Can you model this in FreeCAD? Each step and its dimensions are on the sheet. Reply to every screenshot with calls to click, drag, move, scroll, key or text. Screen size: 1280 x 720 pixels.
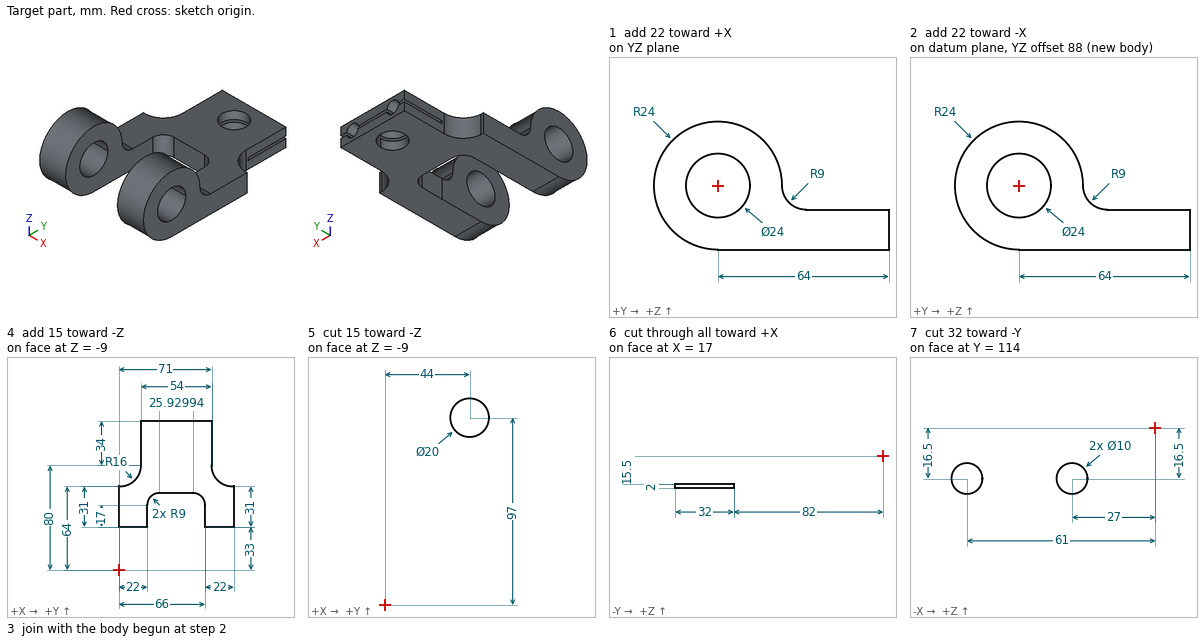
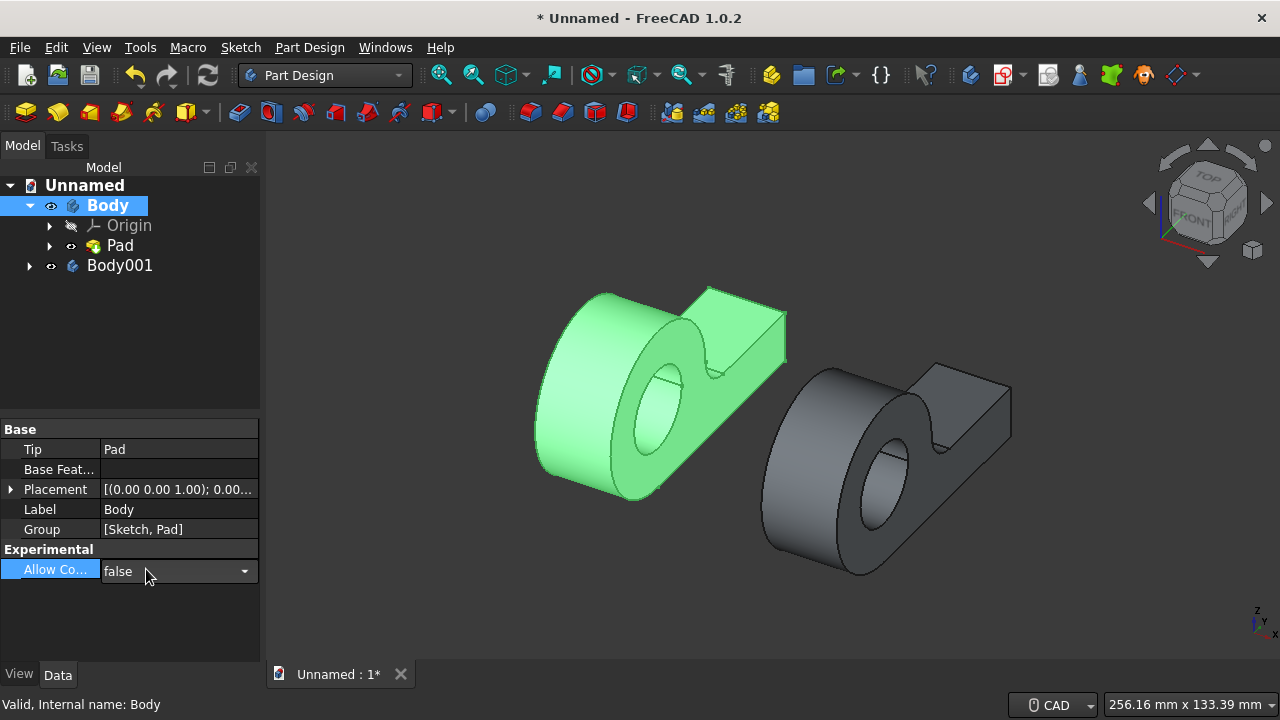
click(146, 569)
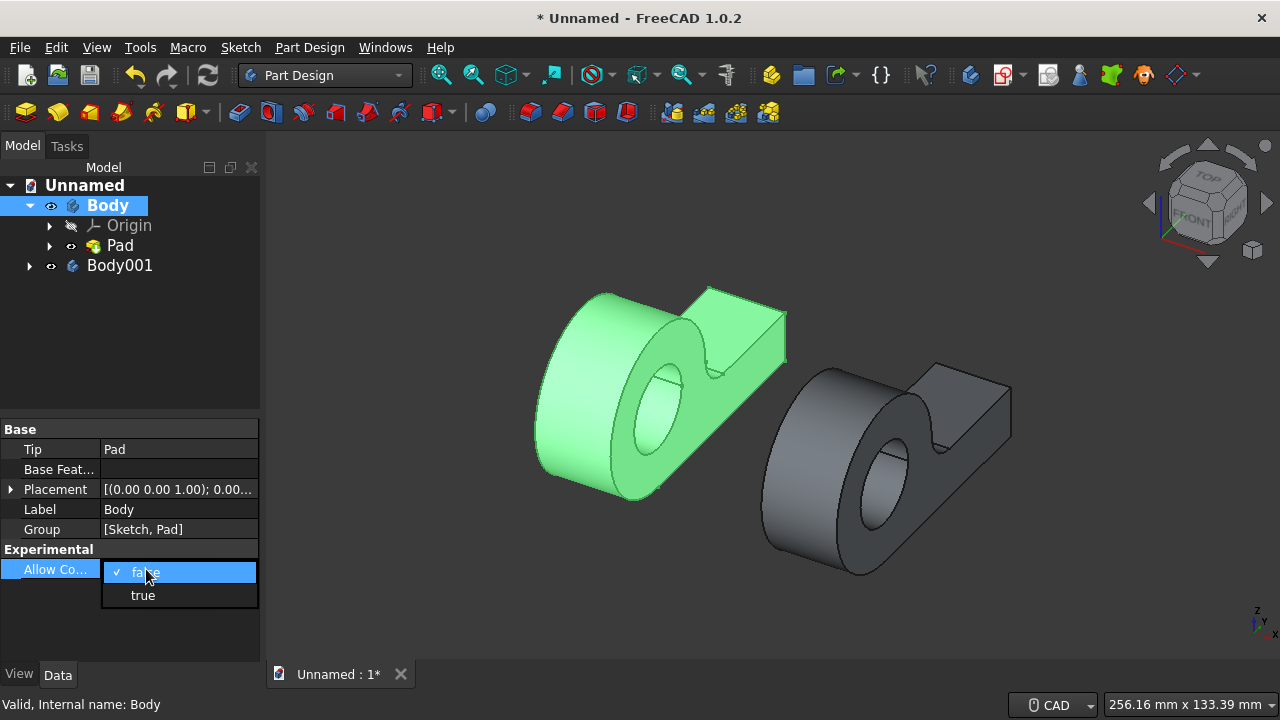
click(179, 596)
key(Return)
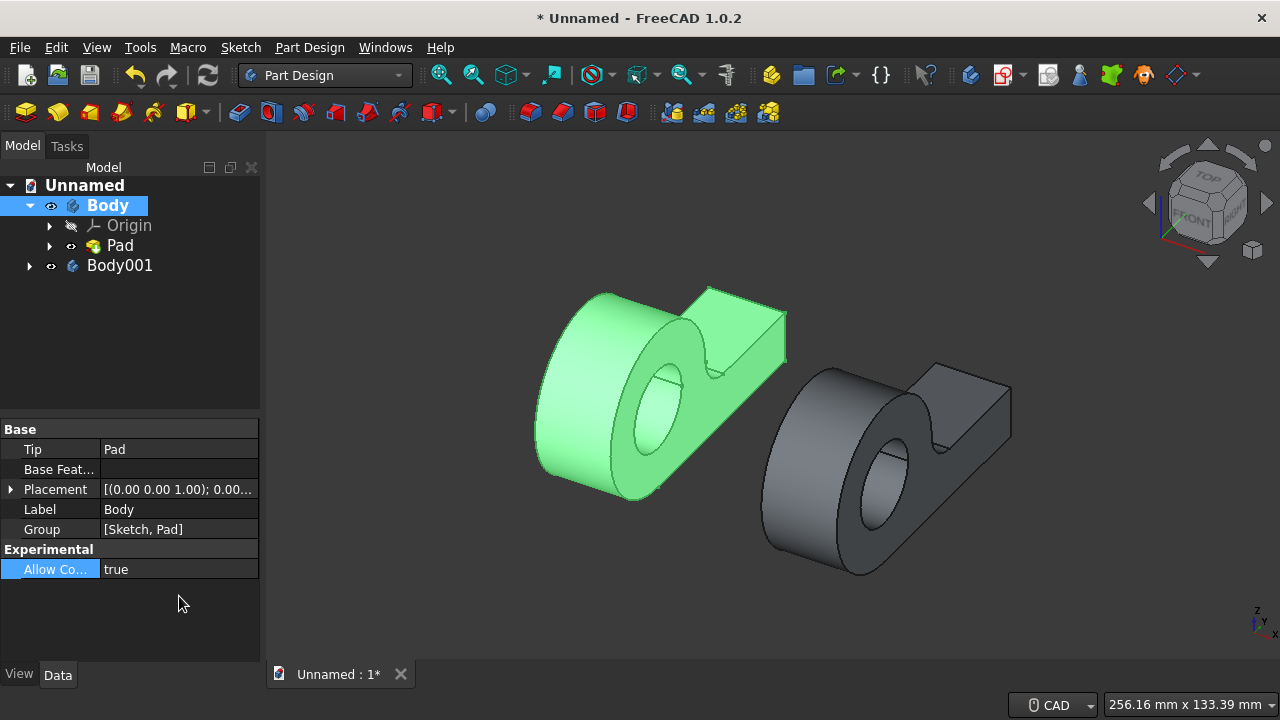
click(96, 266)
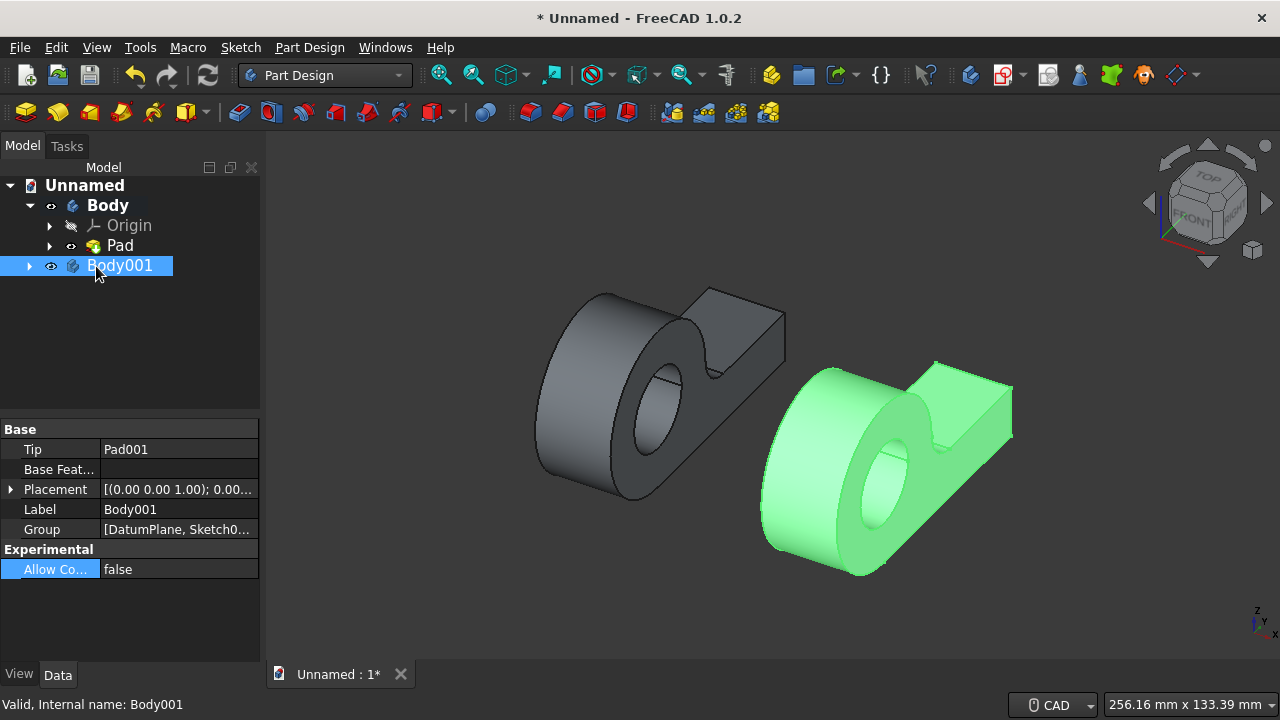
click(486, 112)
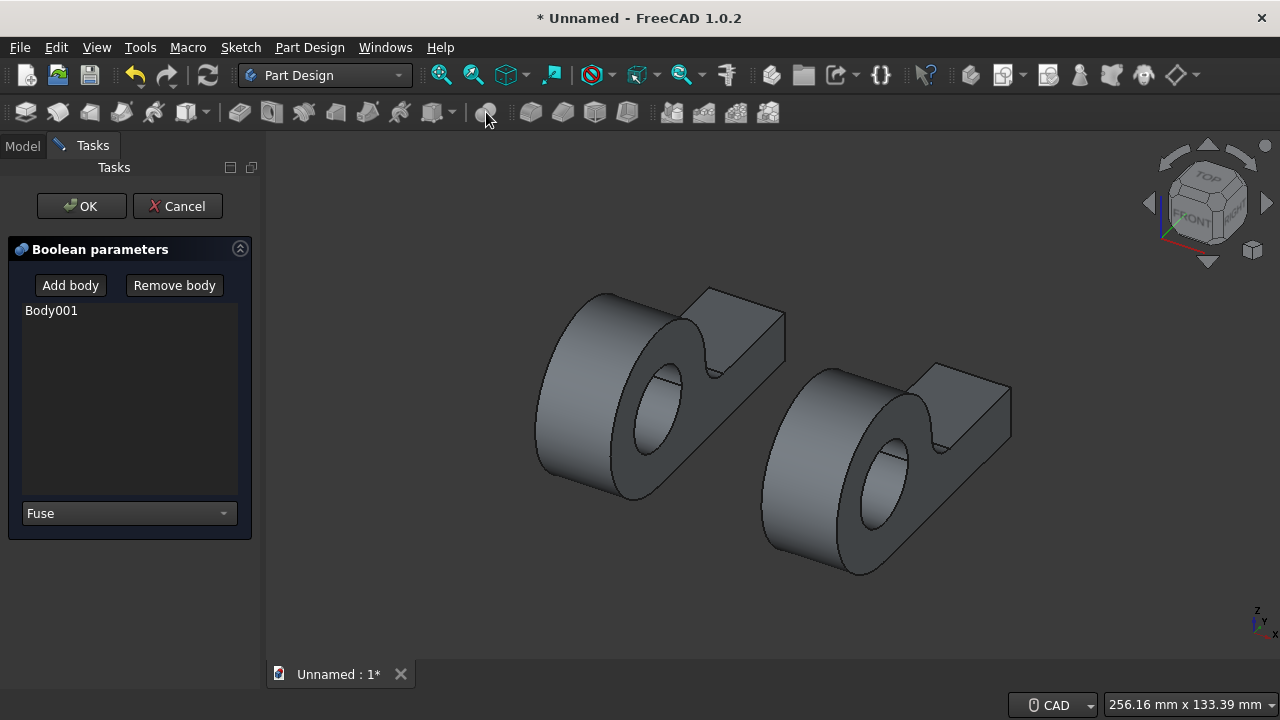
click(82, 206)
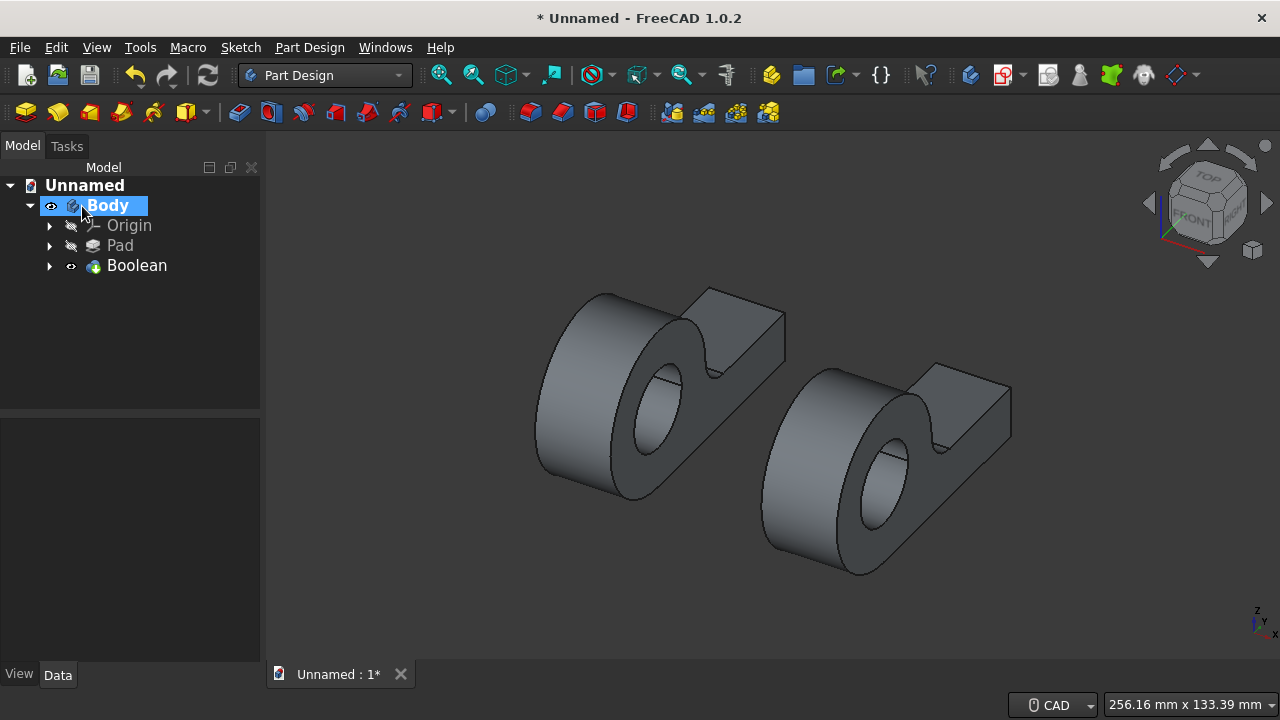
click(725, 321)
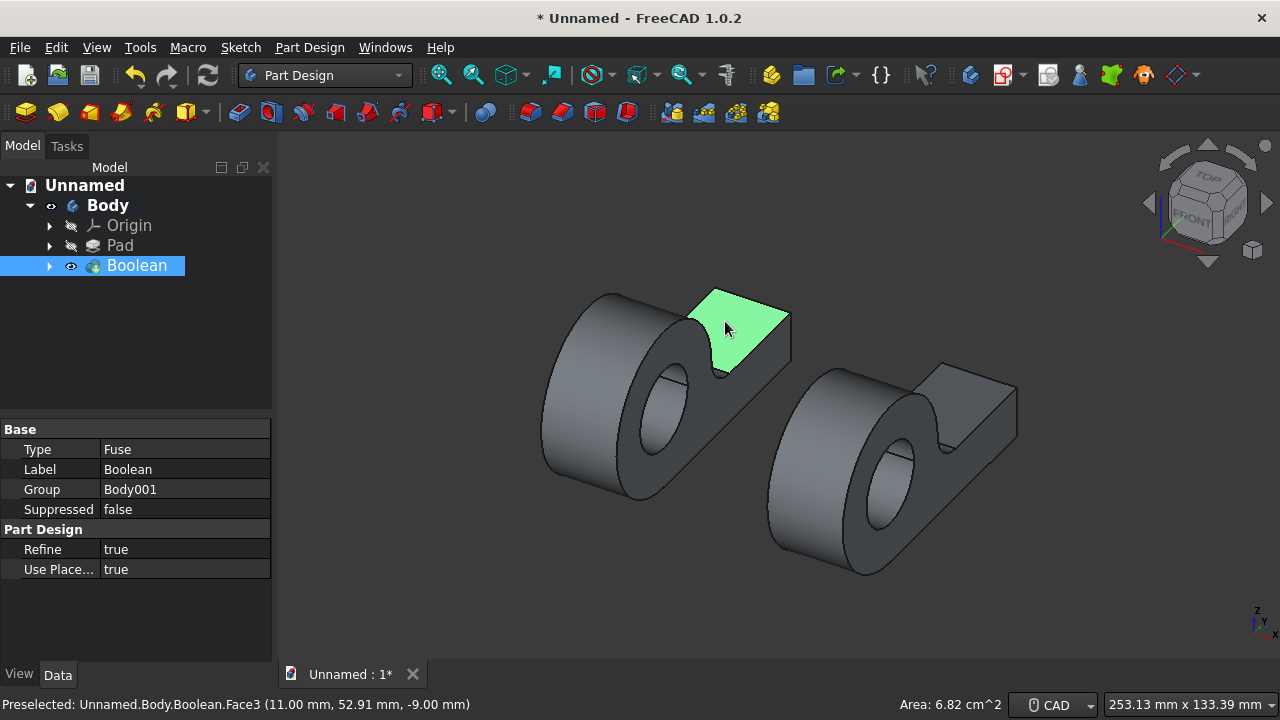
click(1004, 76)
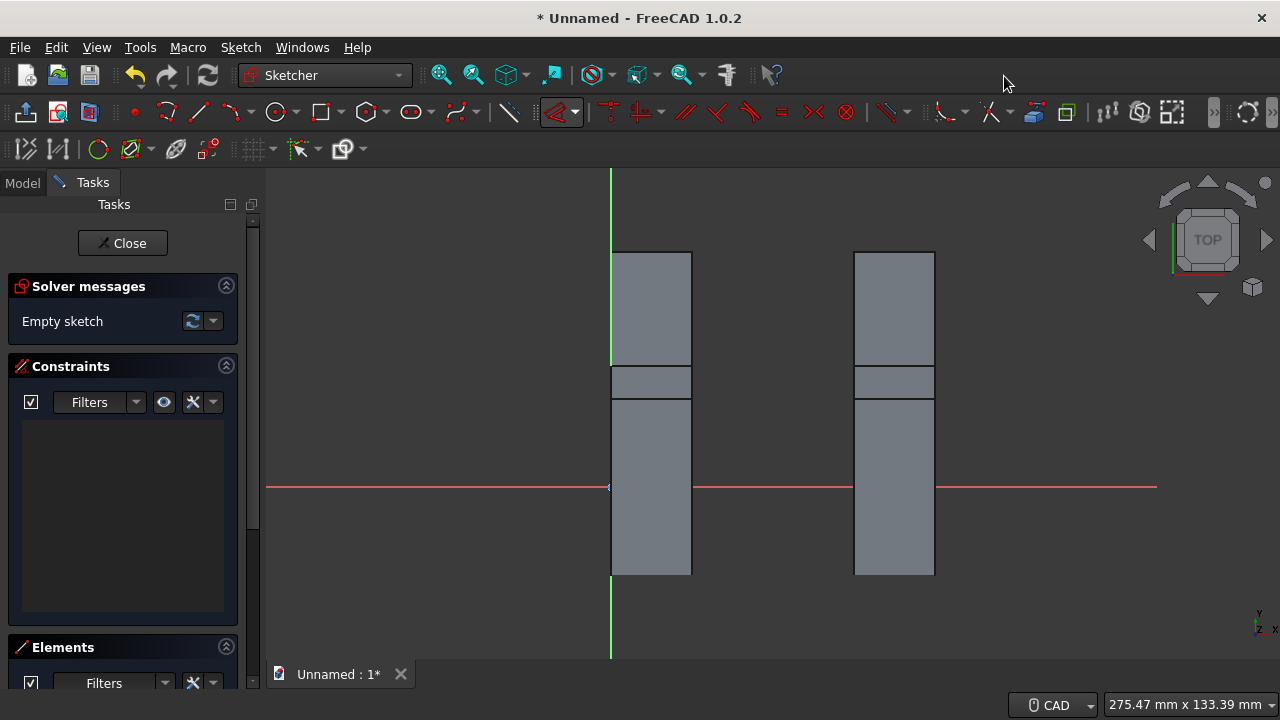
scroll(565, 631, down, 2)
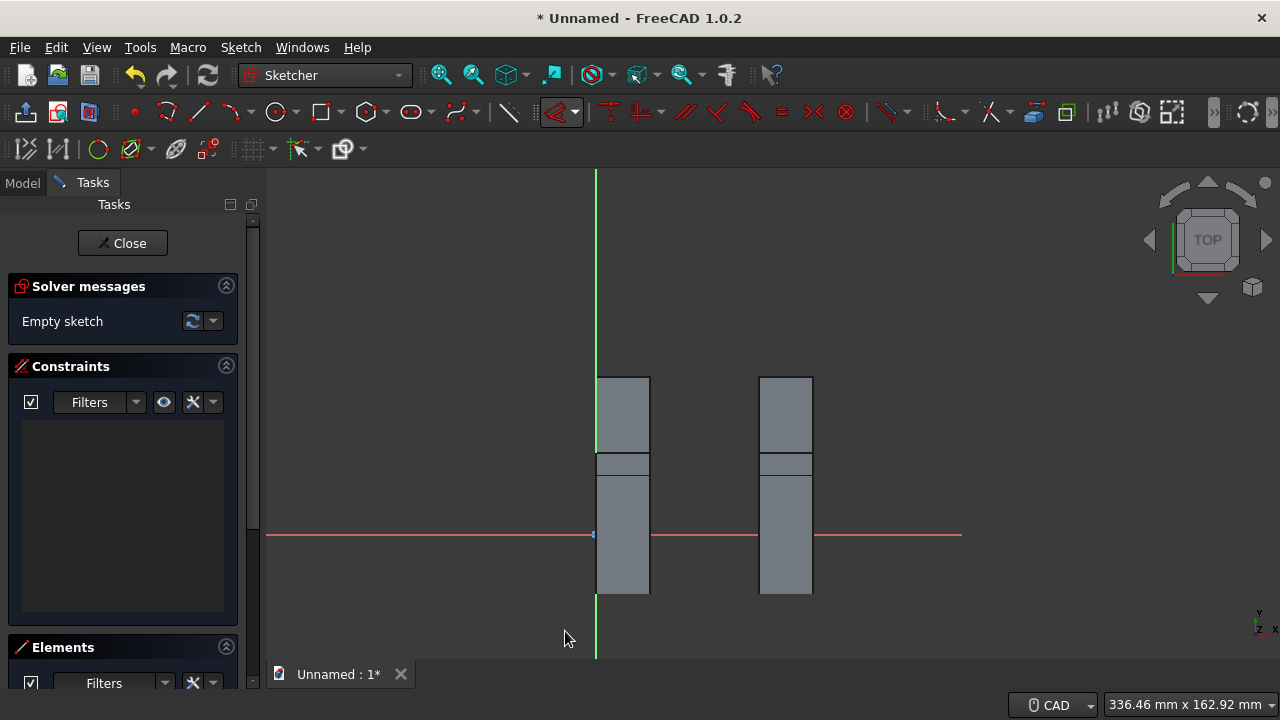
click(168, 112)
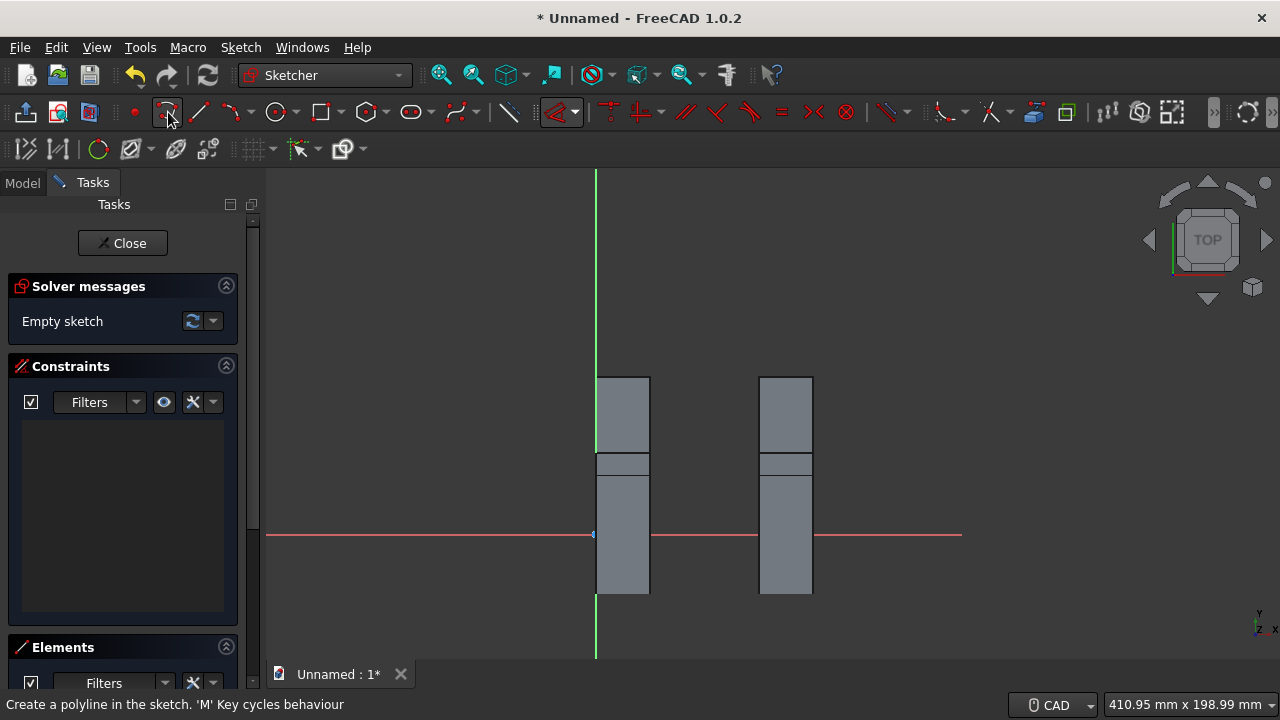
click(596, 377)
click(605, 453)
click(650, 453)
click(650, 411)
right_click(650, 411)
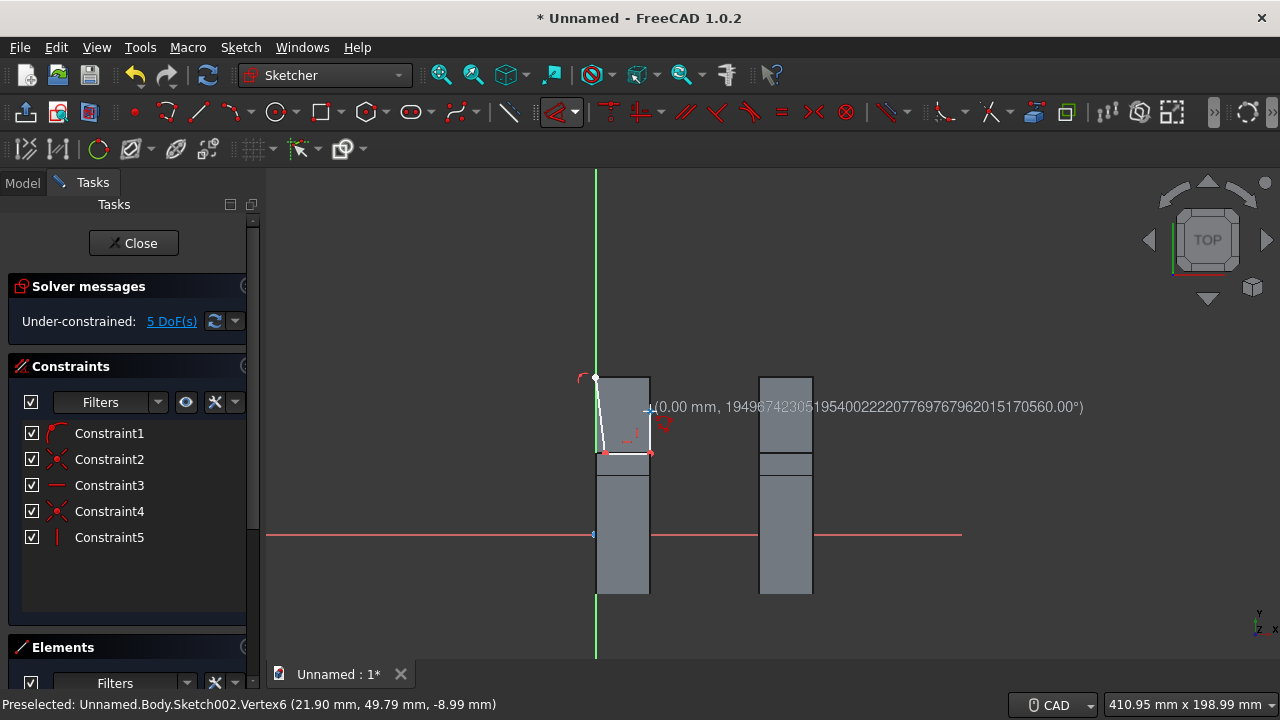
click(200, 112)